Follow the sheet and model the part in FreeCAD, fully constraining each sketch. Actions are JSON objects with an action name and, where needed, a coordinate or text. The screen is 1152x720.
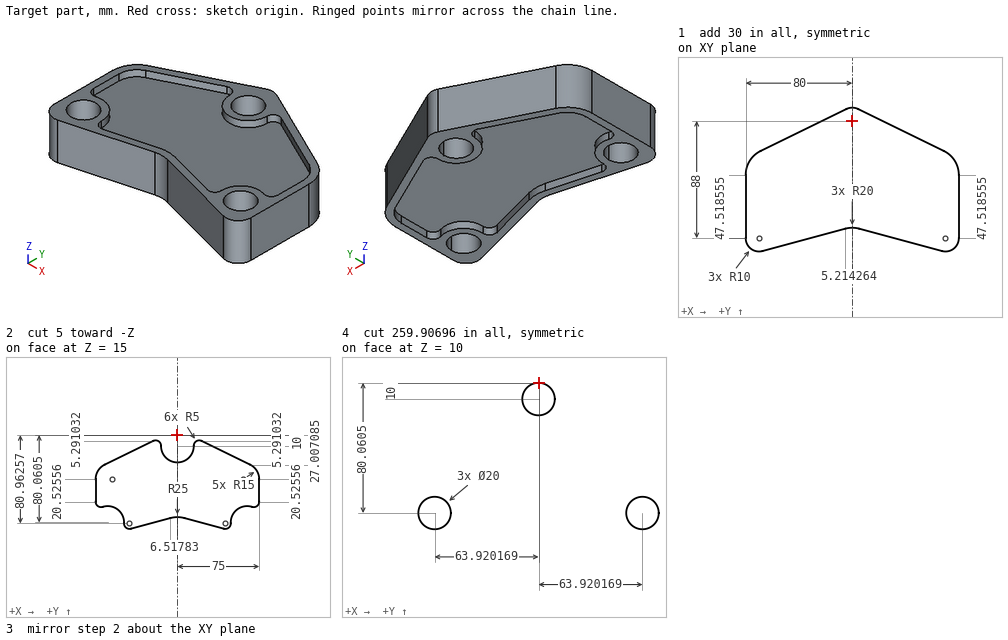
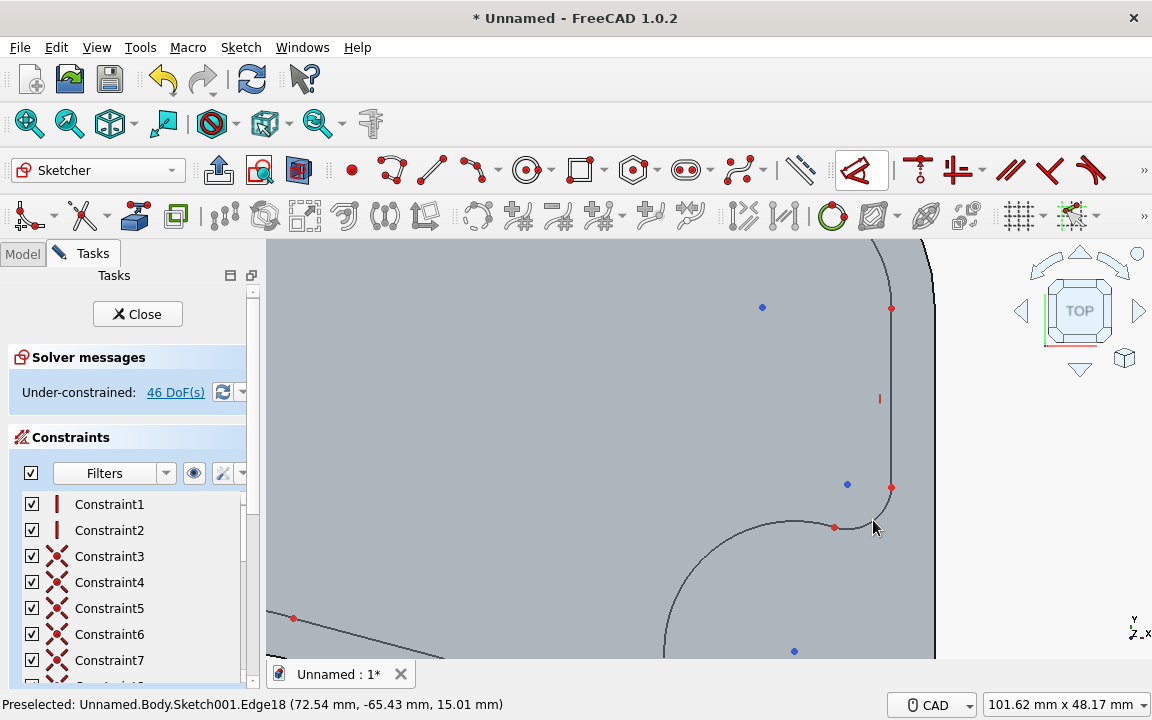
{"action": "left_click", "coordinate": [891, 434]}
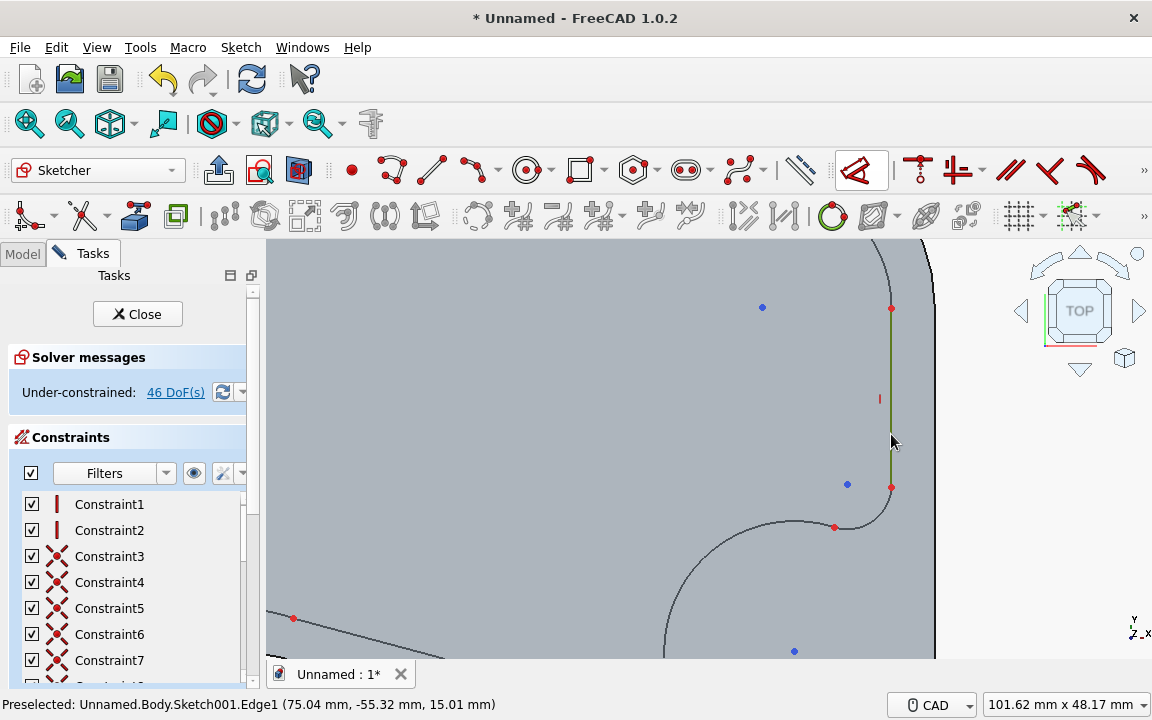
{"action": "left_click", "coordinate": [888, 280]}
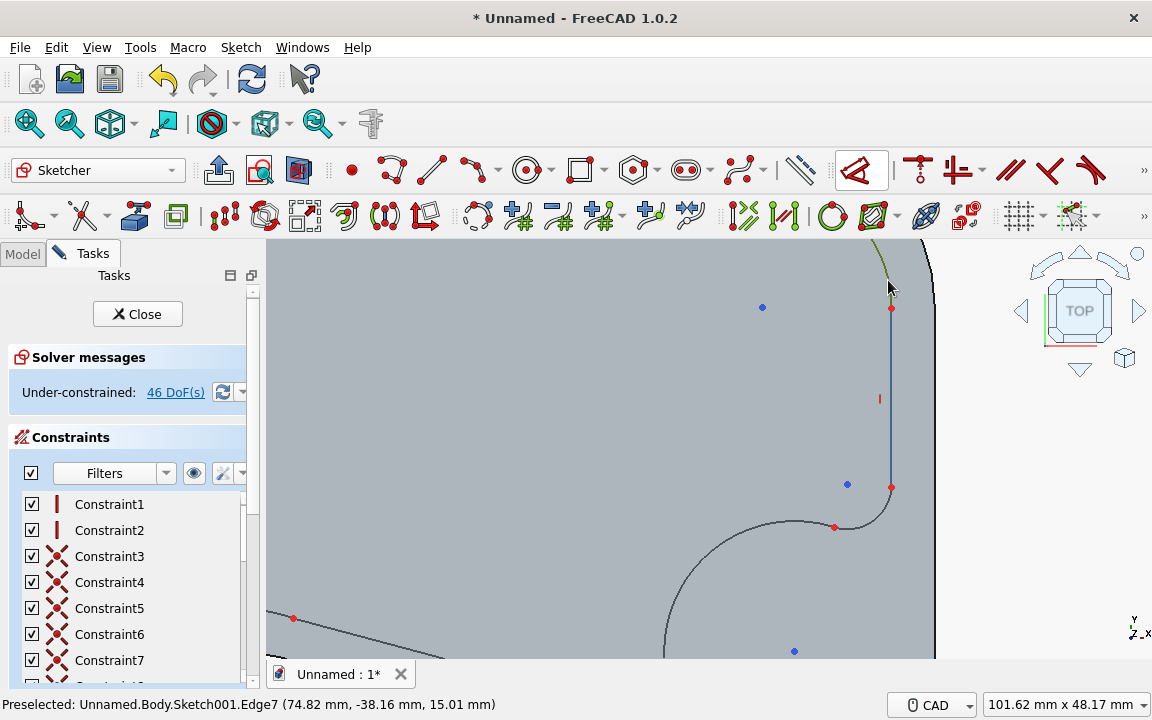
{"action": "key", "text": "t"}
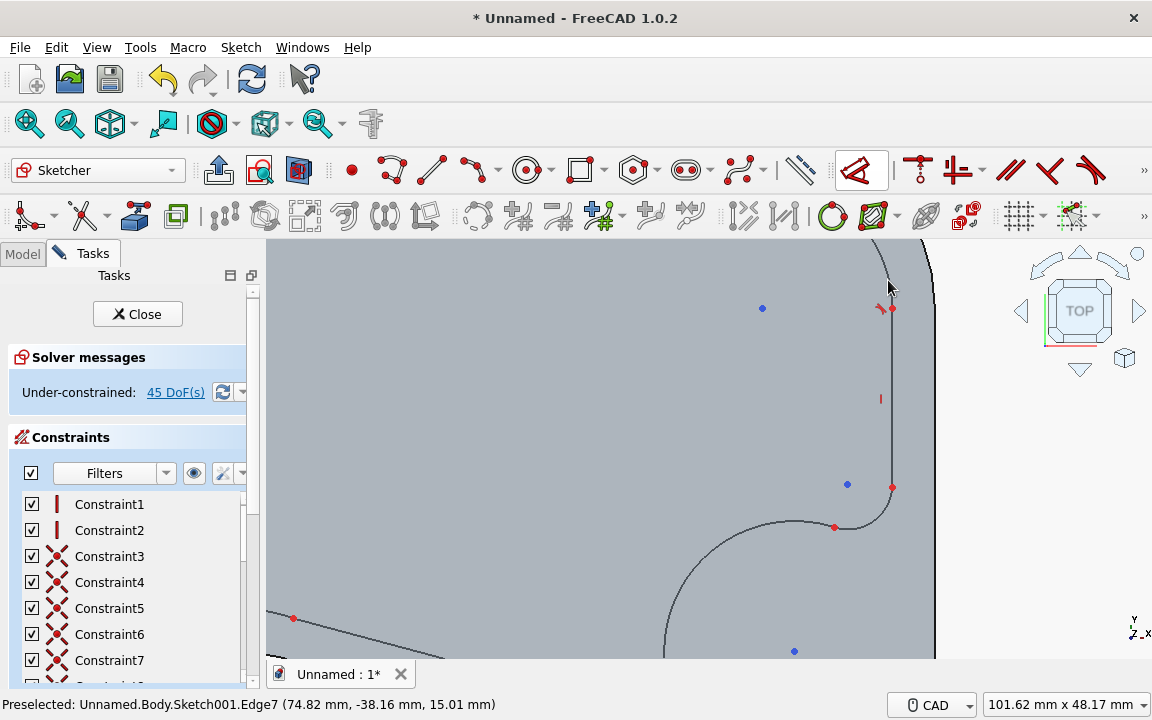
{"action": "left_click", "coordinate": [892, 434]}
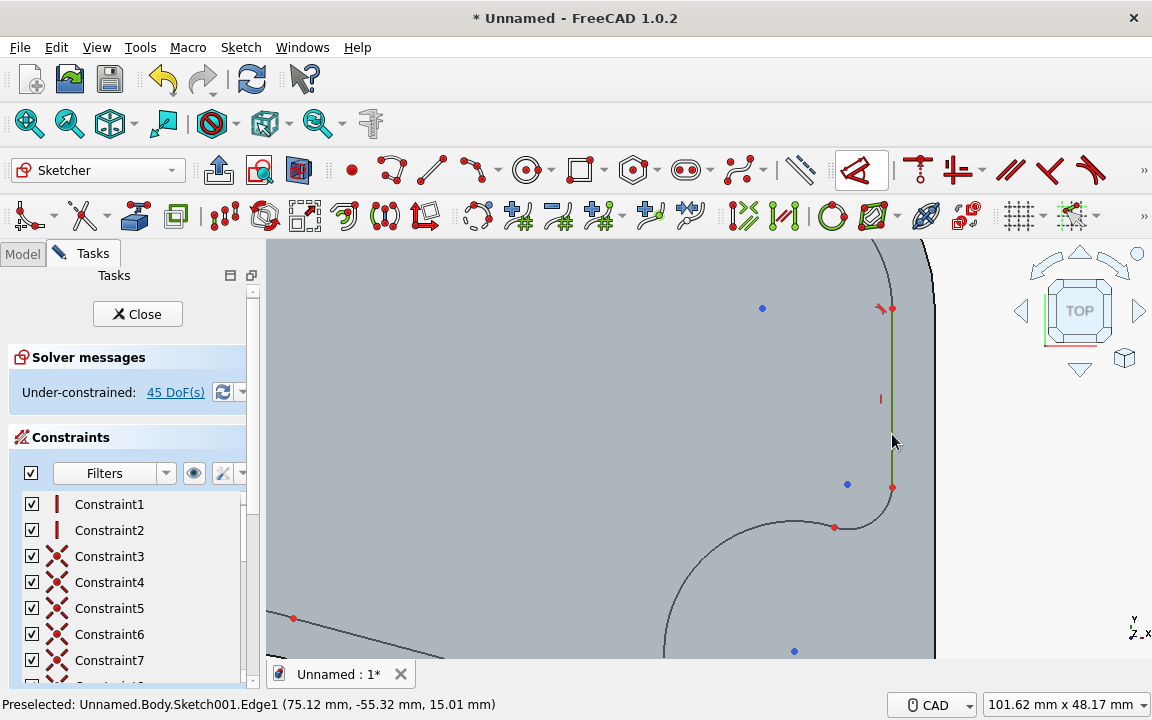
{"action": "left_click", "coordinate": [858, 528]}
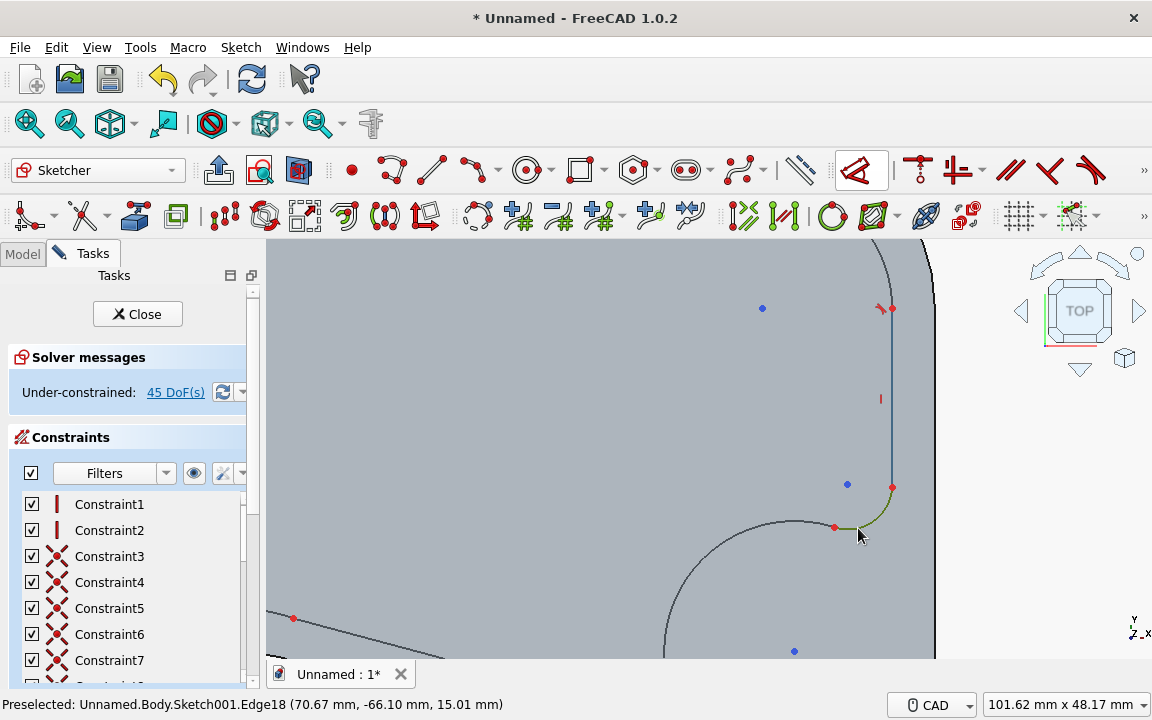
{"action": "left_click", "coordinate": [1092, 170]}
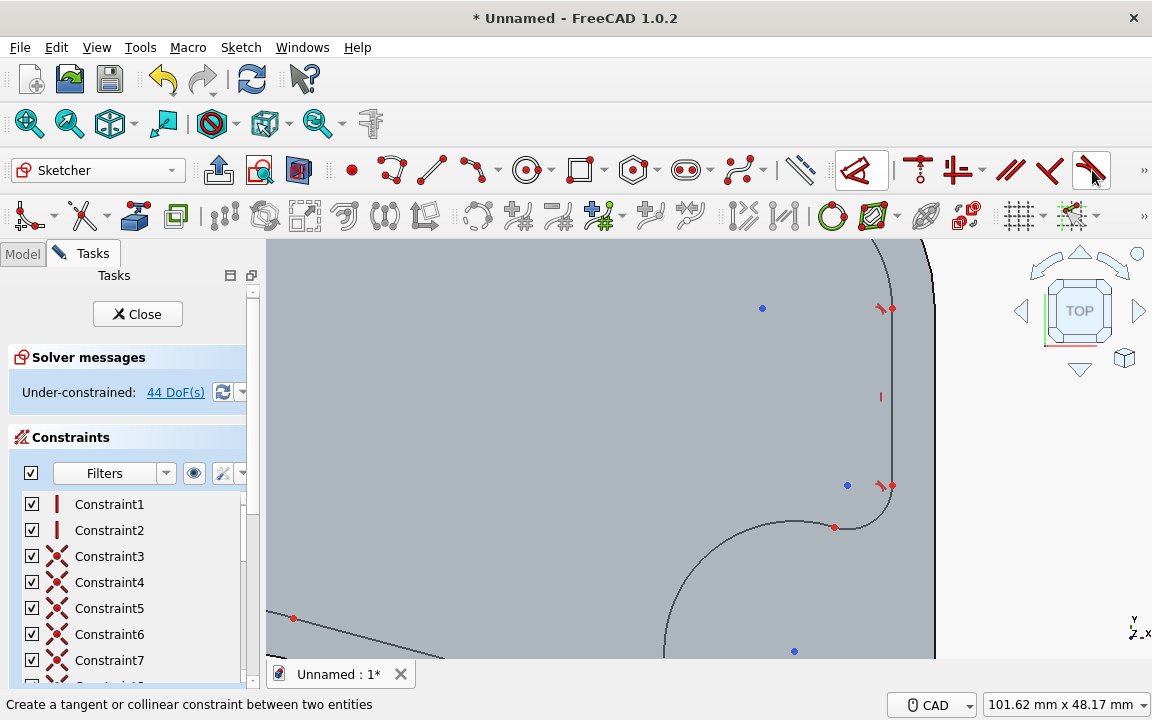
{"action": "scroll", "coordinate": [875, 520], "scroll_direction": "down", "scroll_amount": 5}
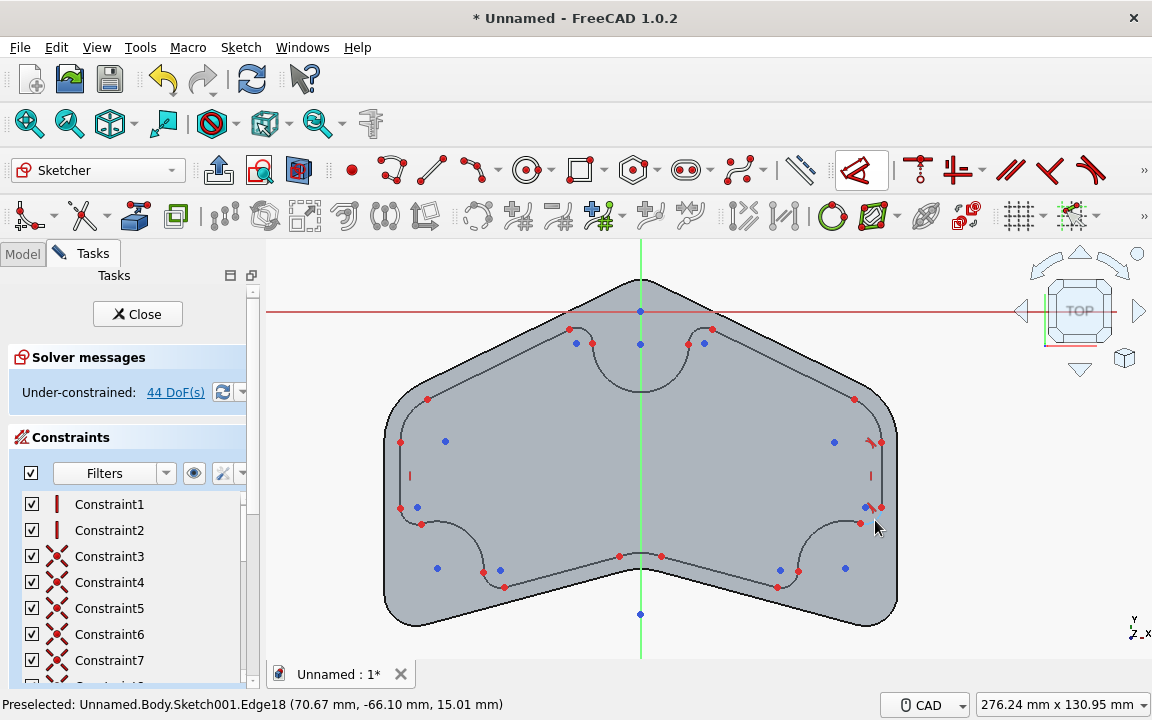
{"action": "left_click", "coordinate": [812, 379]}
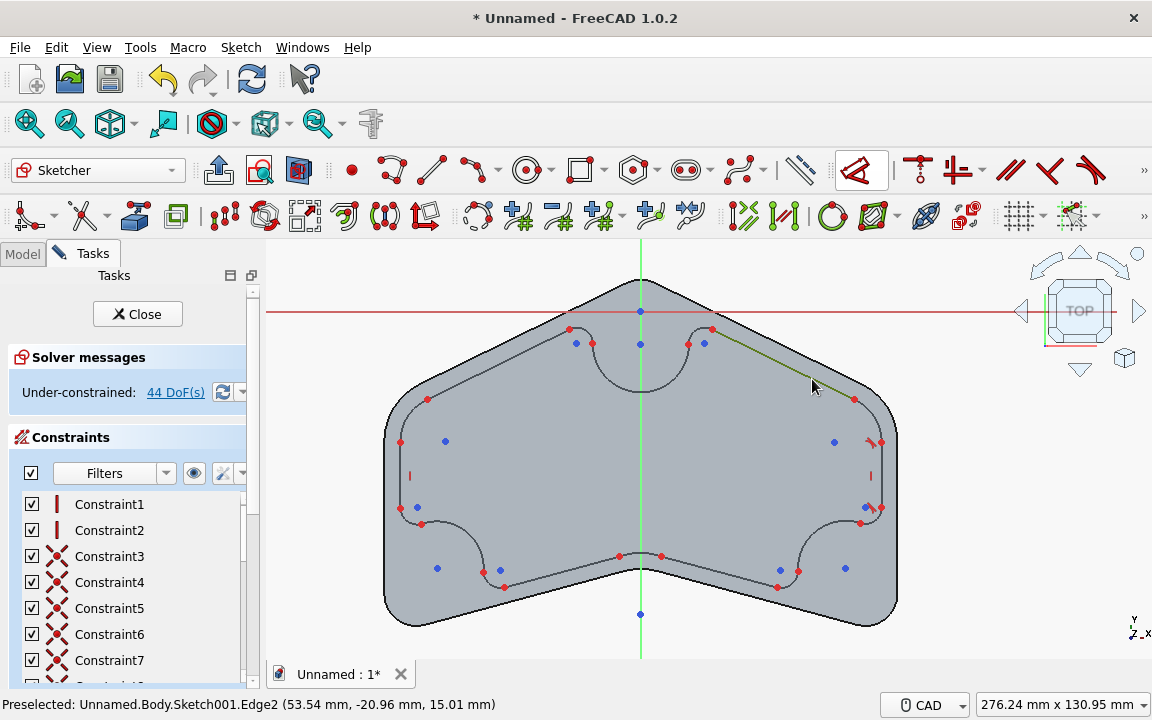
{"action": "left_click", "coordinate": [879, 427]}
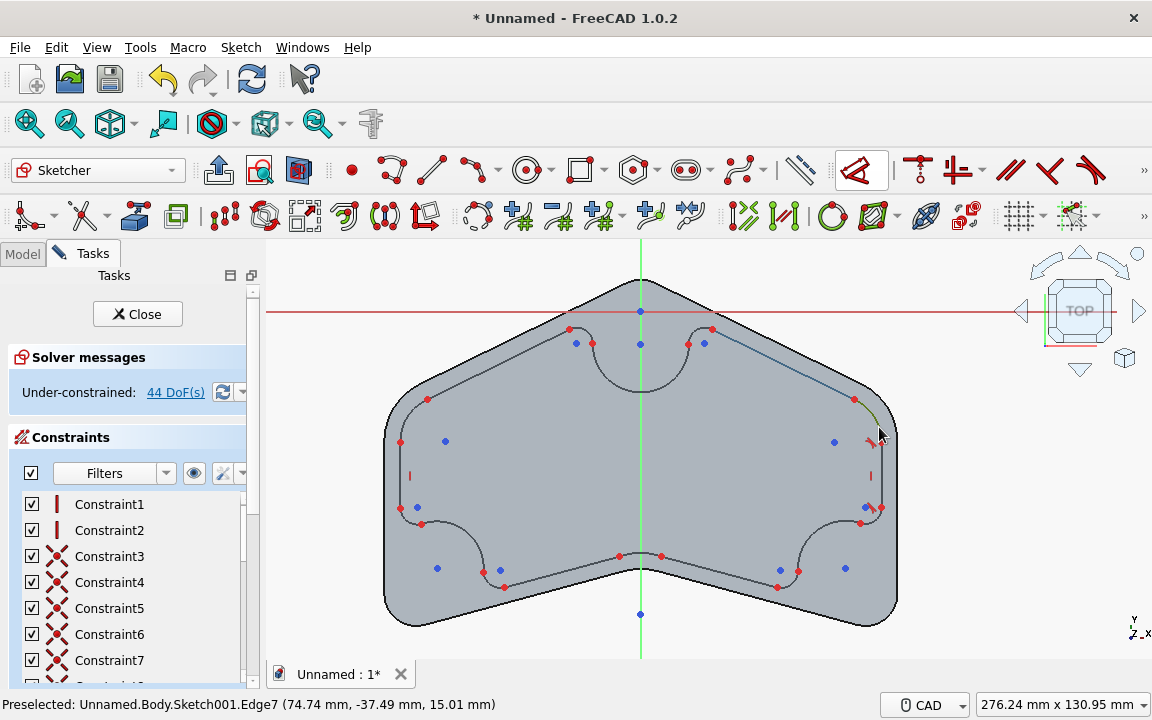
{"action": "key", "text": "t"}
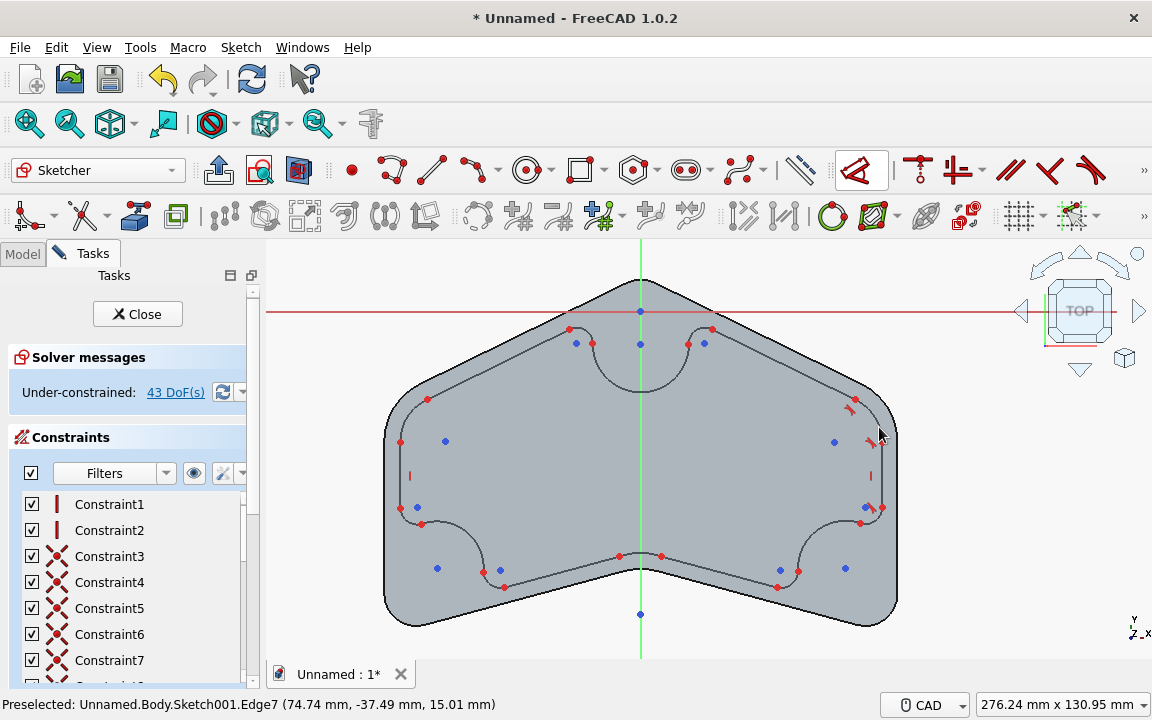
{"action": "left_click", "coordinate": [812, 379]}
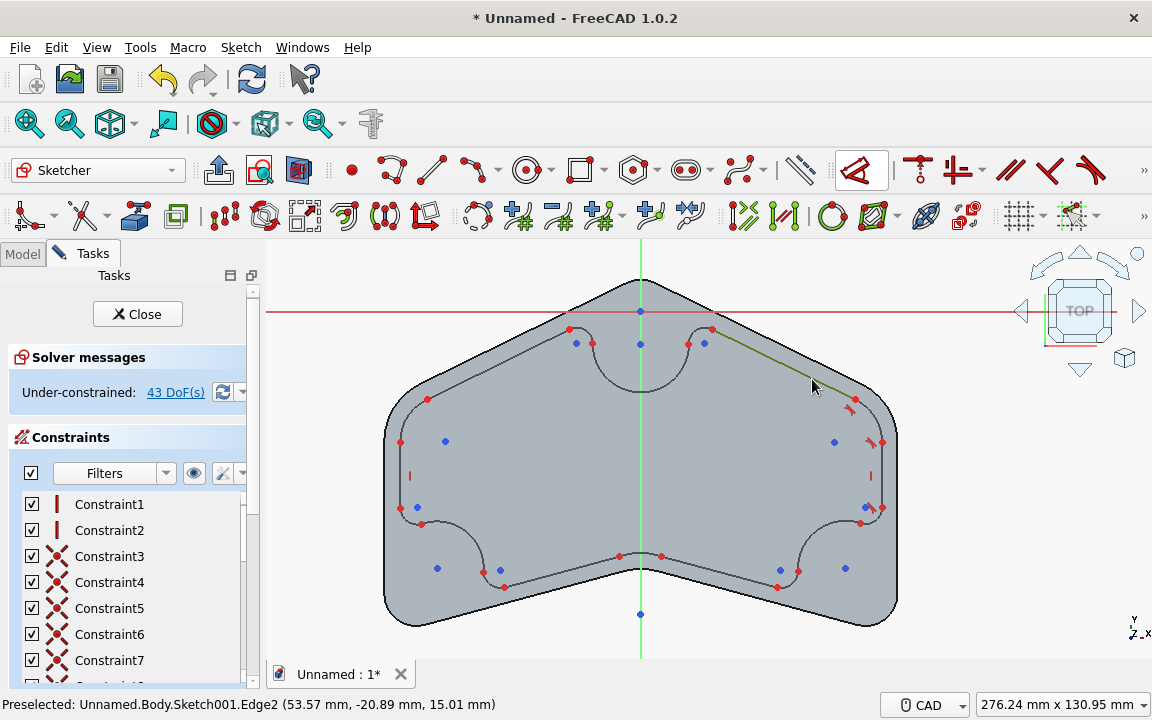
{"action": "scroll", "coordinate": [703, 328], "scroll_direction": "up", "scroll_amount": 2}